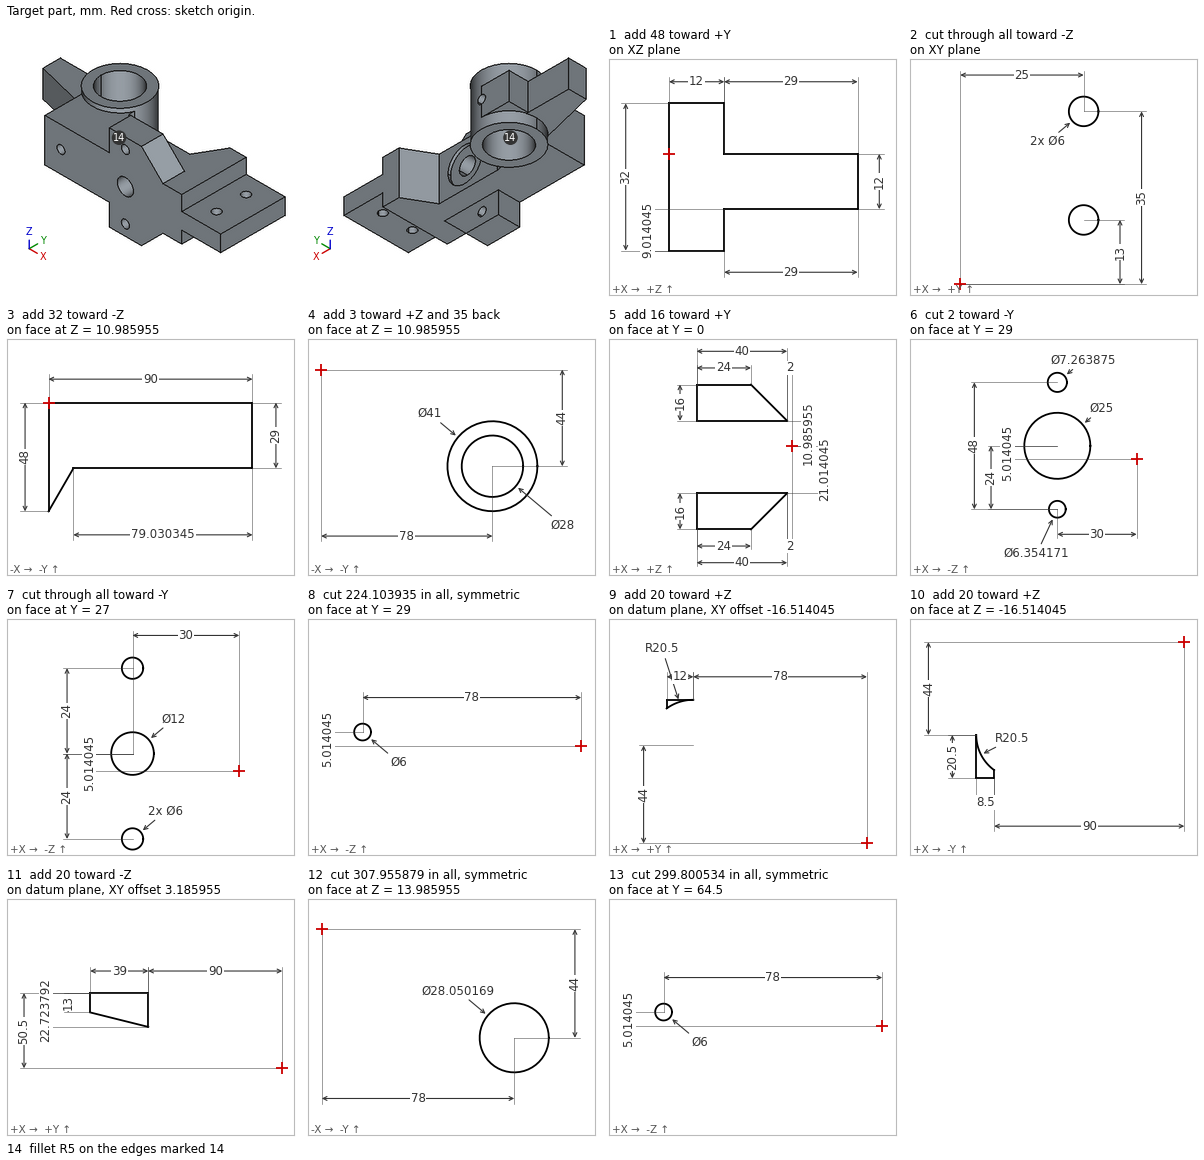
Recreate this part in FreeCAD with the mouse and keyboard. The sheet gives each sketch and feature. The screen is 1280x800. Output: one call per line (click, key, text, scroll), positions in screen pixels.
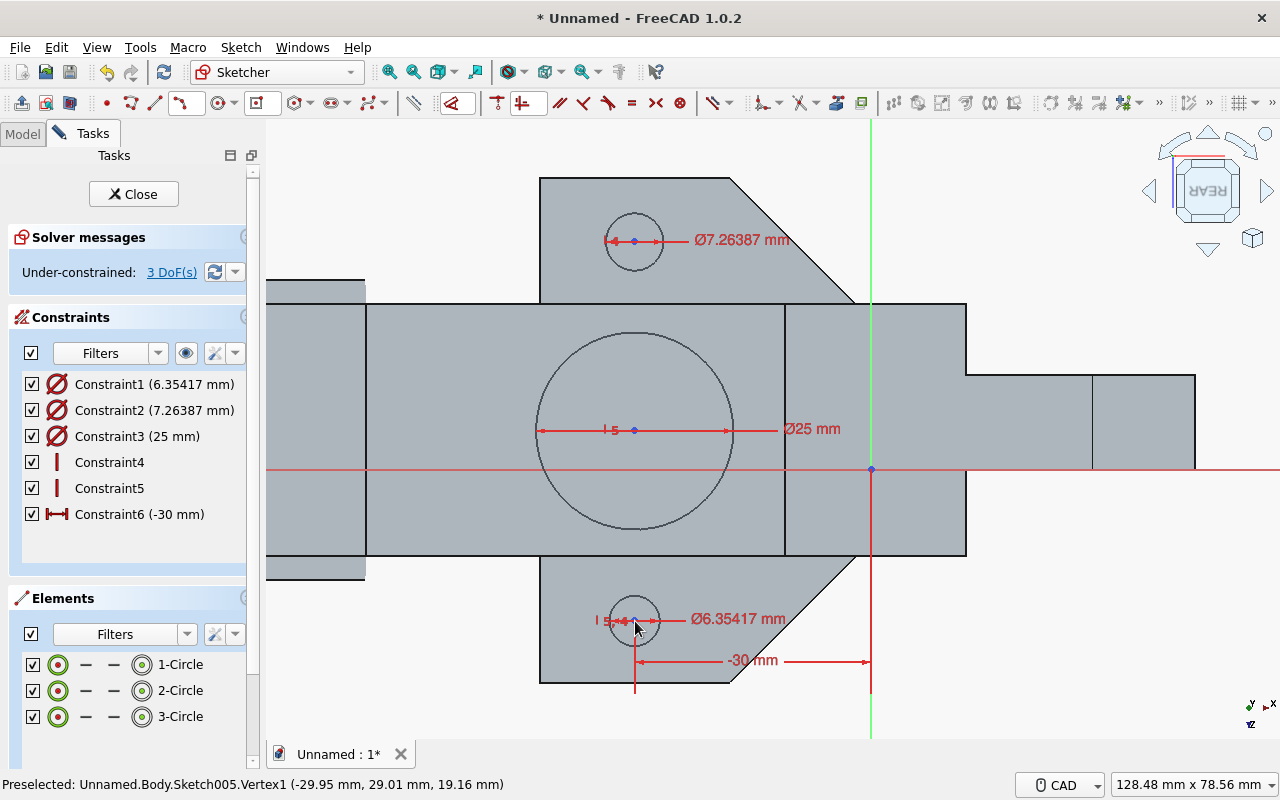
click(635, 621)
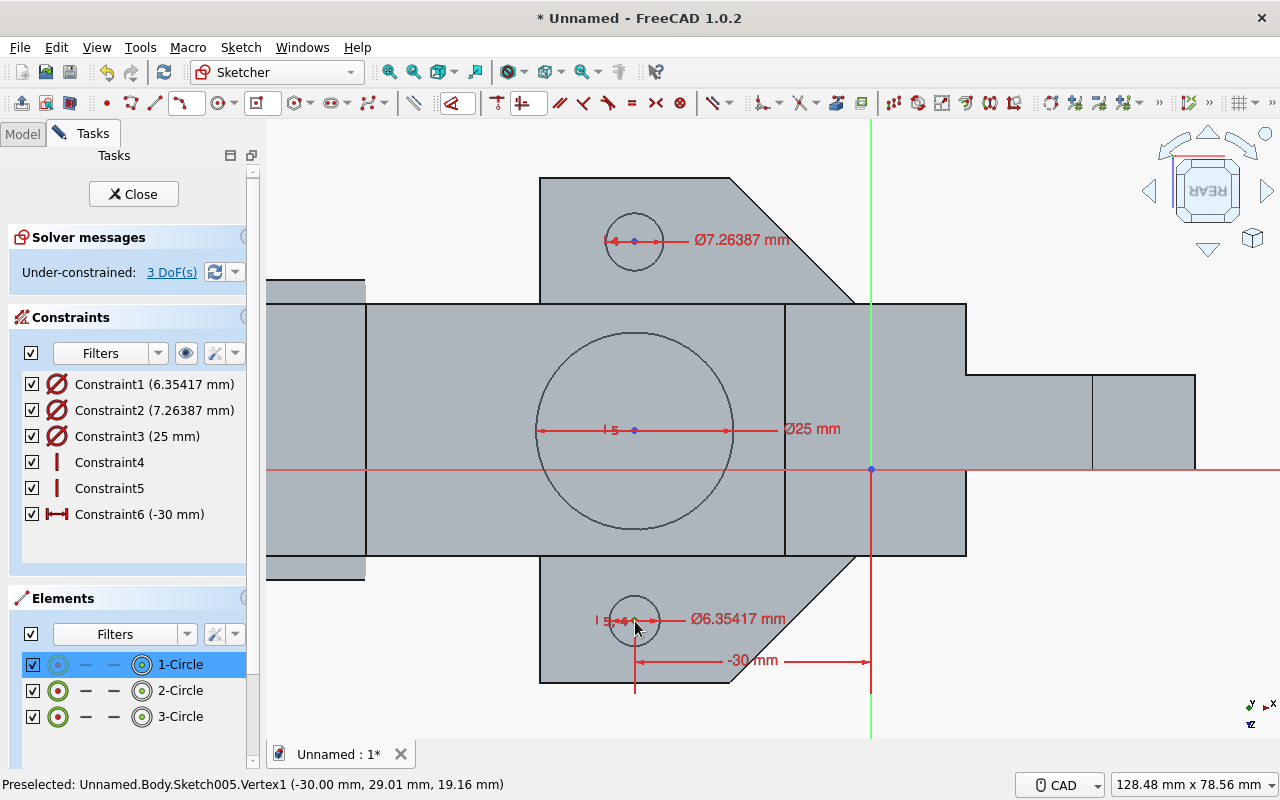
click(635, 242)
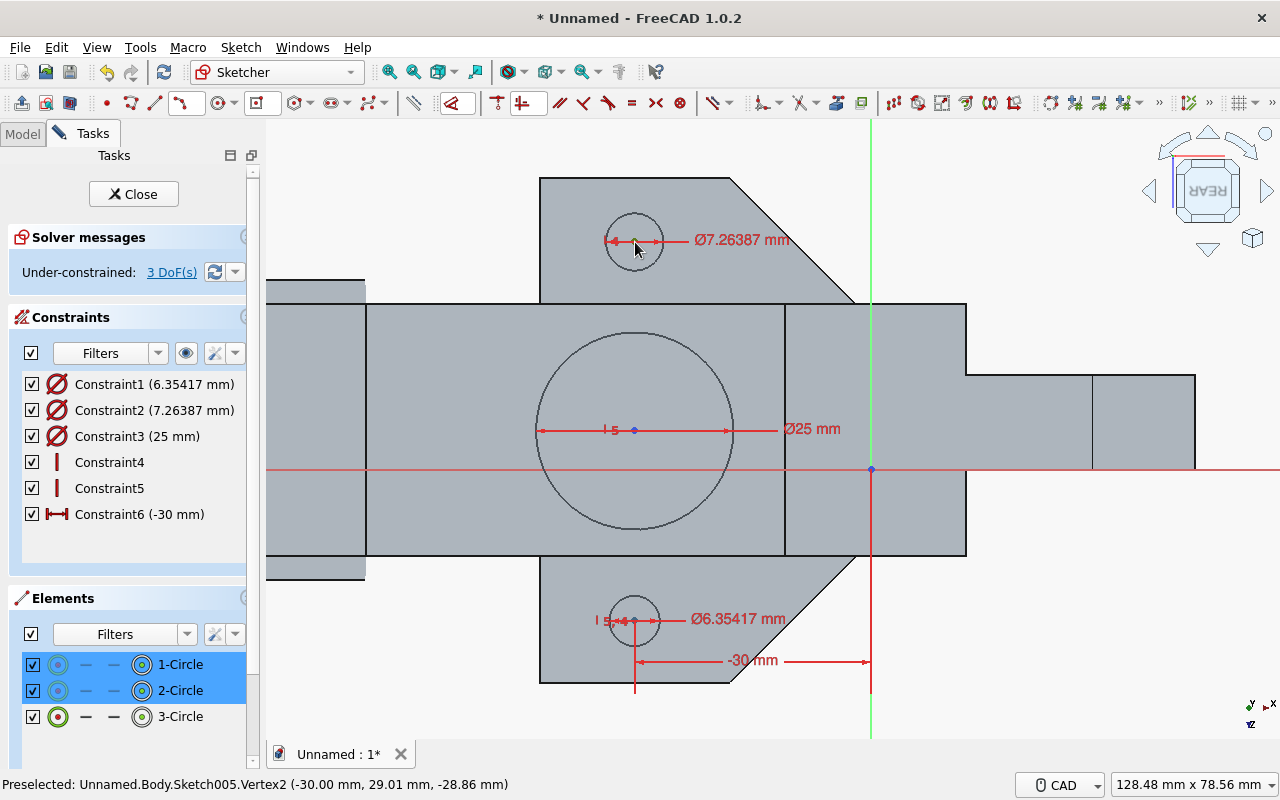
key(i)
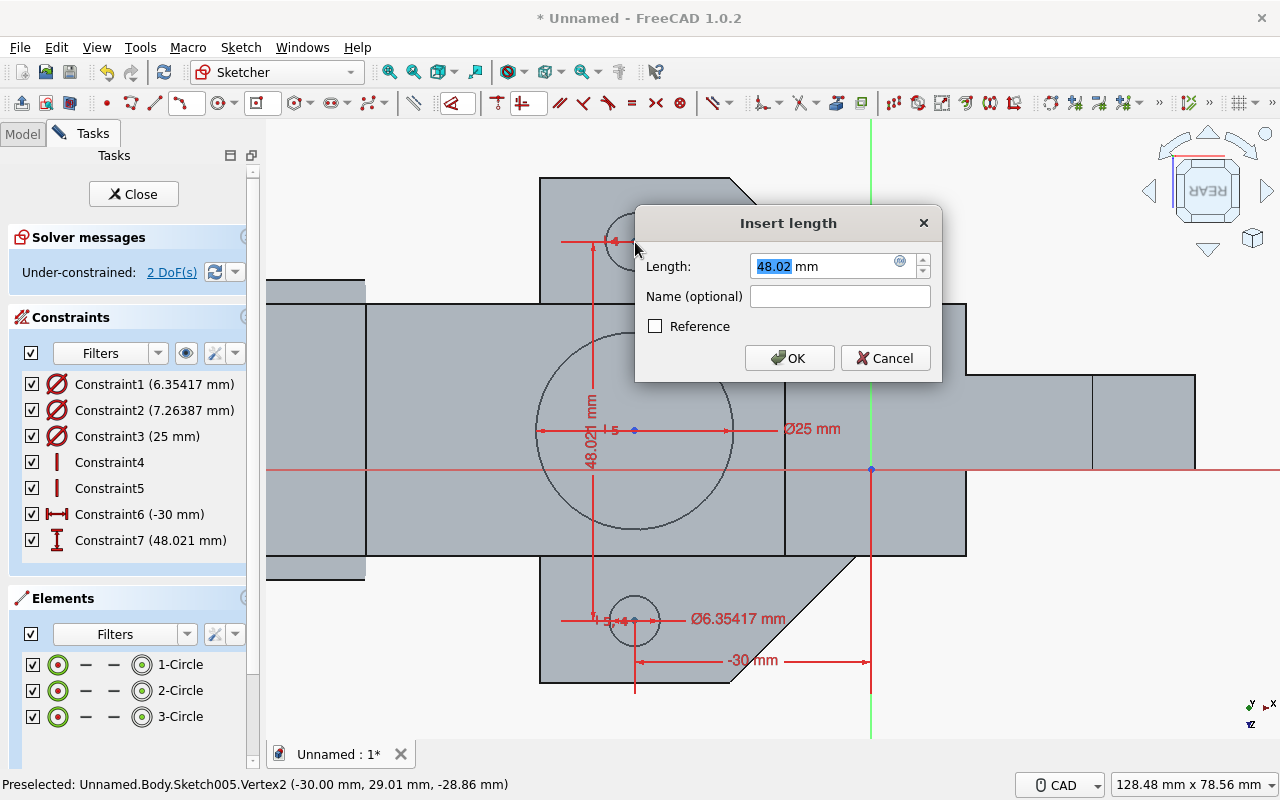
text(48)
key(Return)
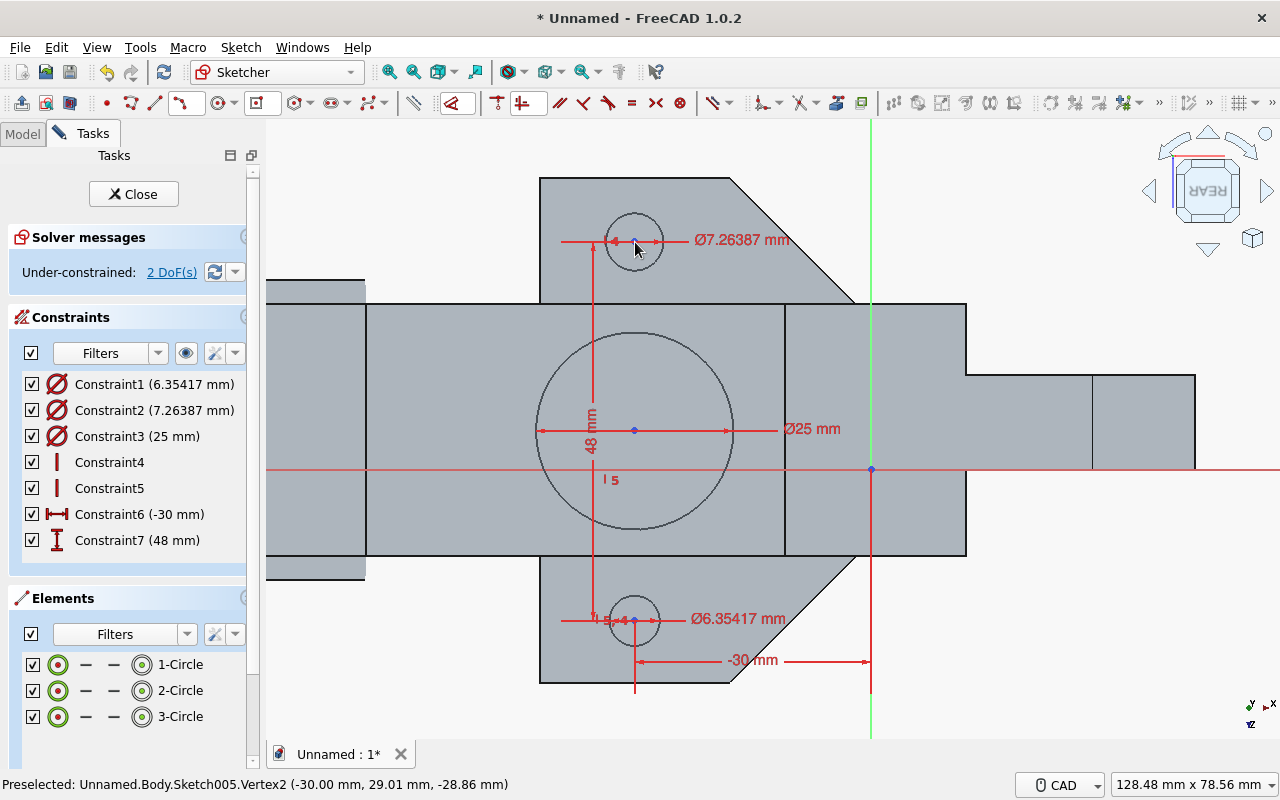
click(635, 621)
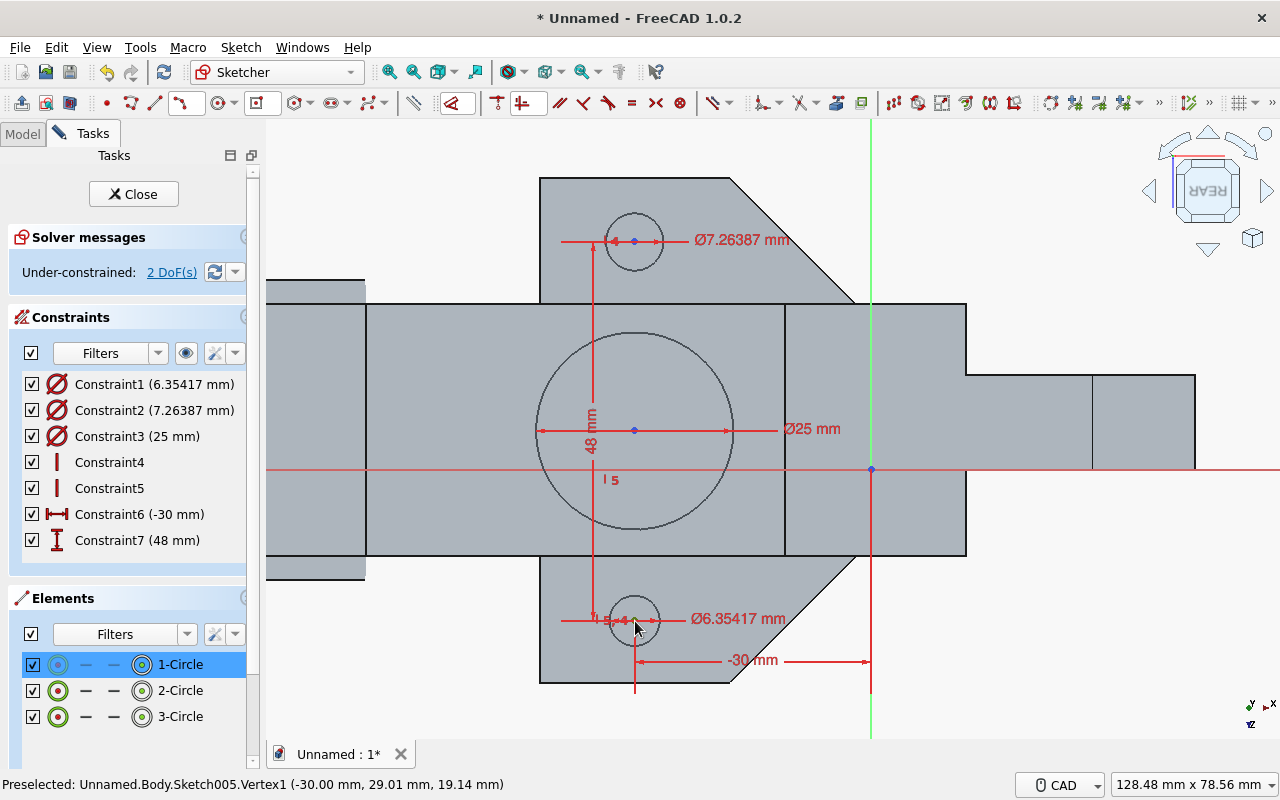
click(635, 431)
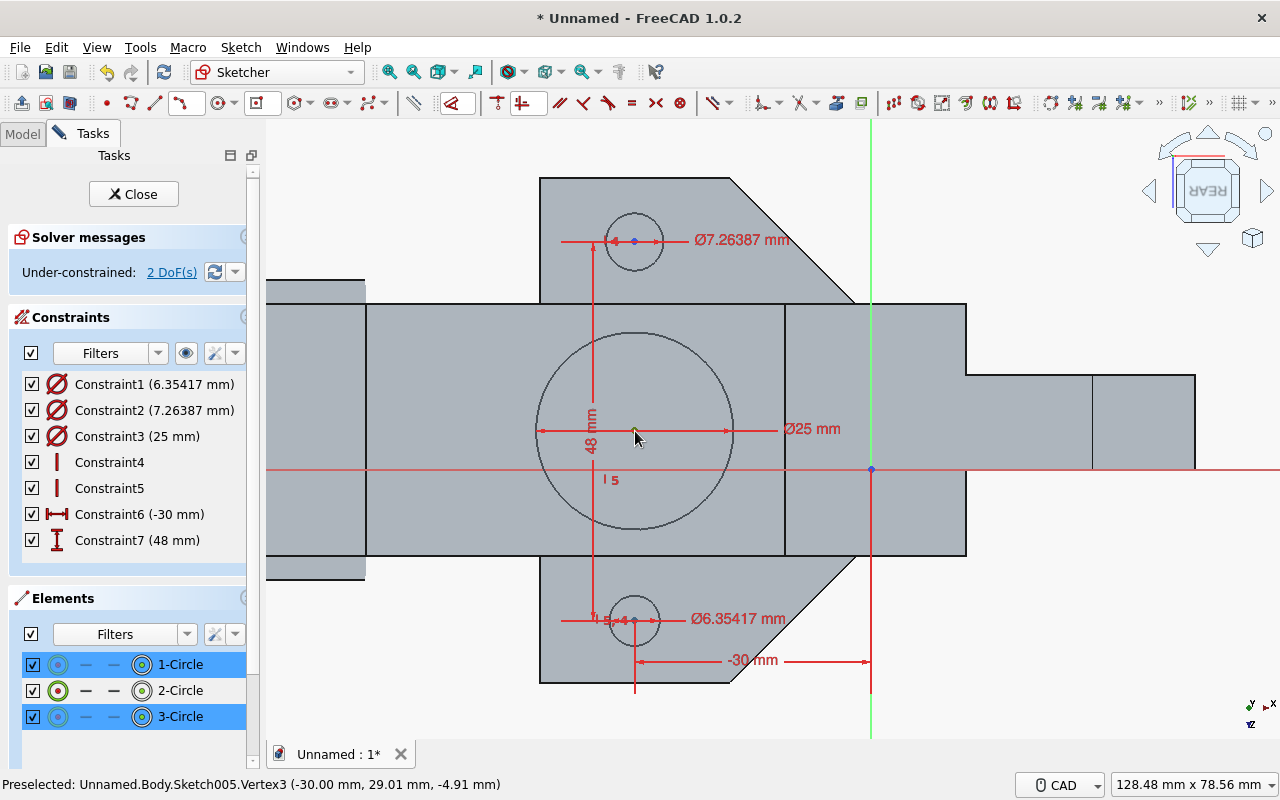
click(470, 104)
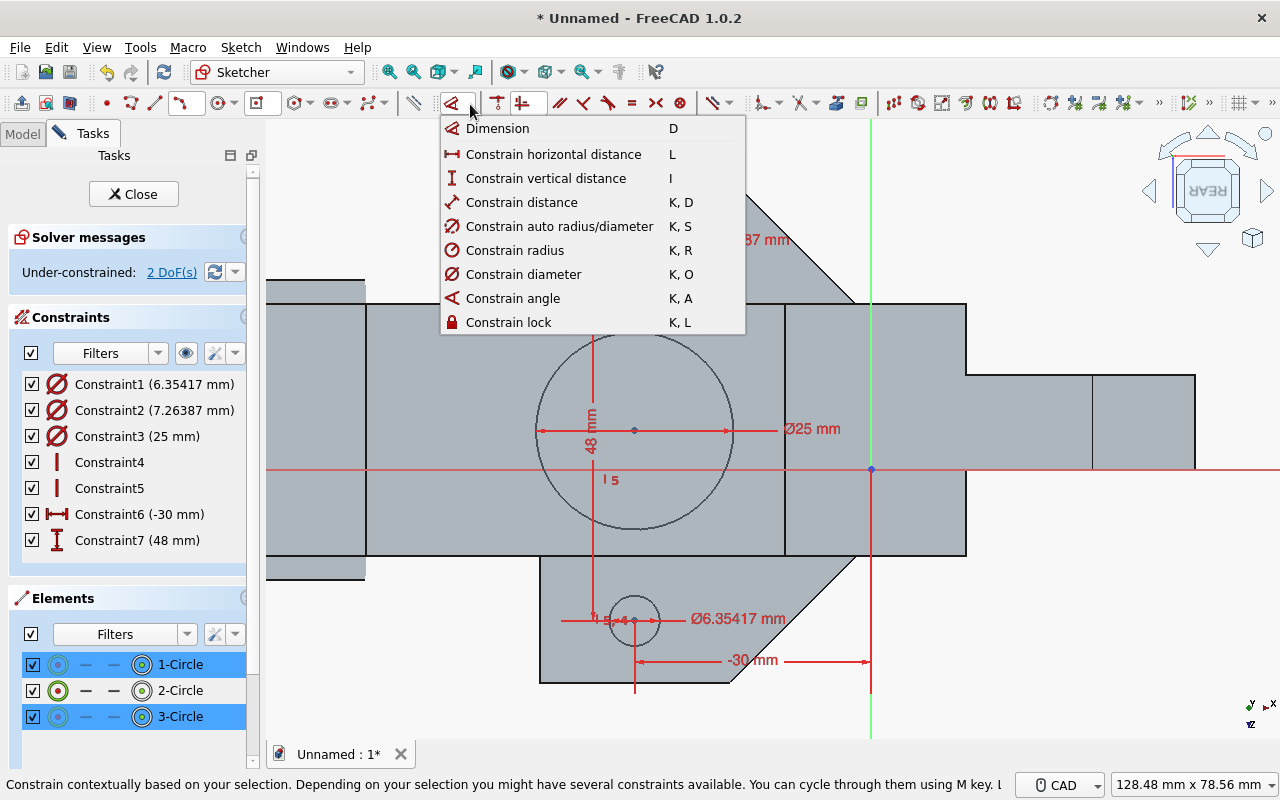
click(593, 178)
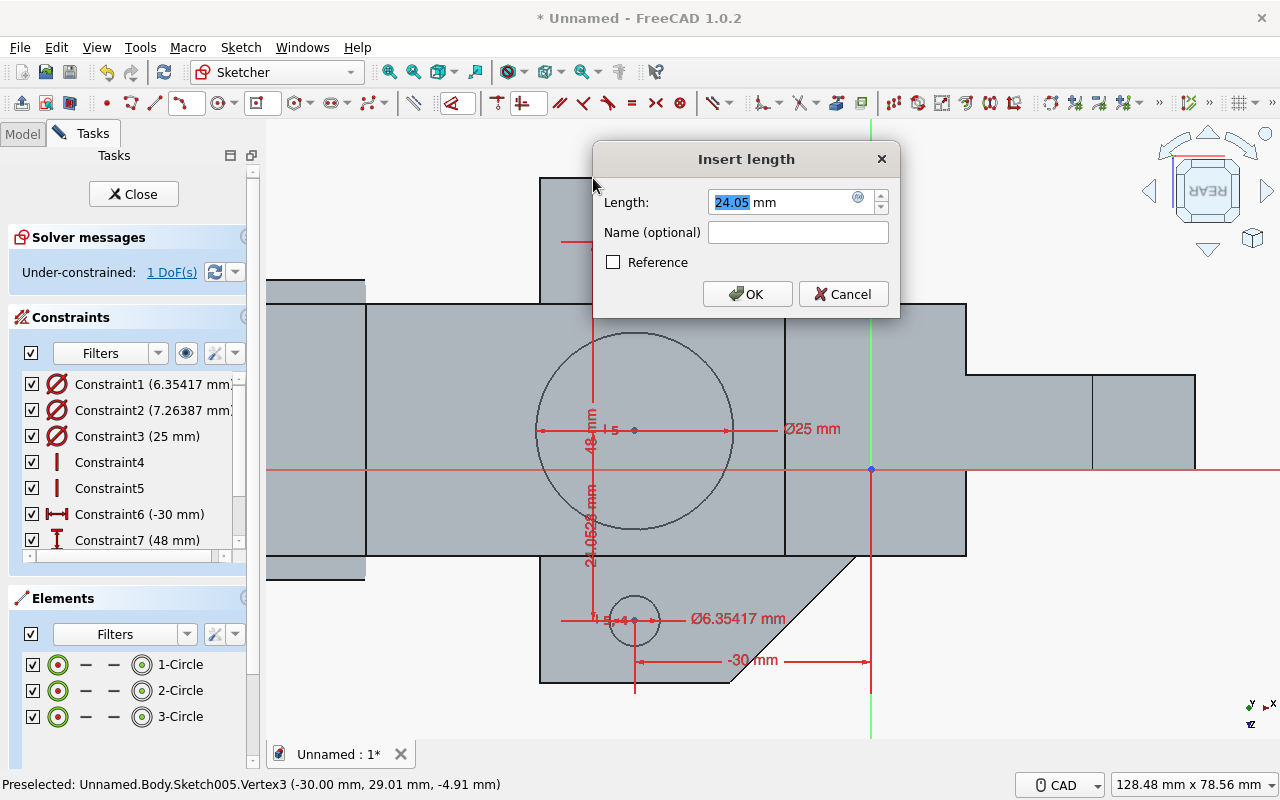
text(24)
key(Return)